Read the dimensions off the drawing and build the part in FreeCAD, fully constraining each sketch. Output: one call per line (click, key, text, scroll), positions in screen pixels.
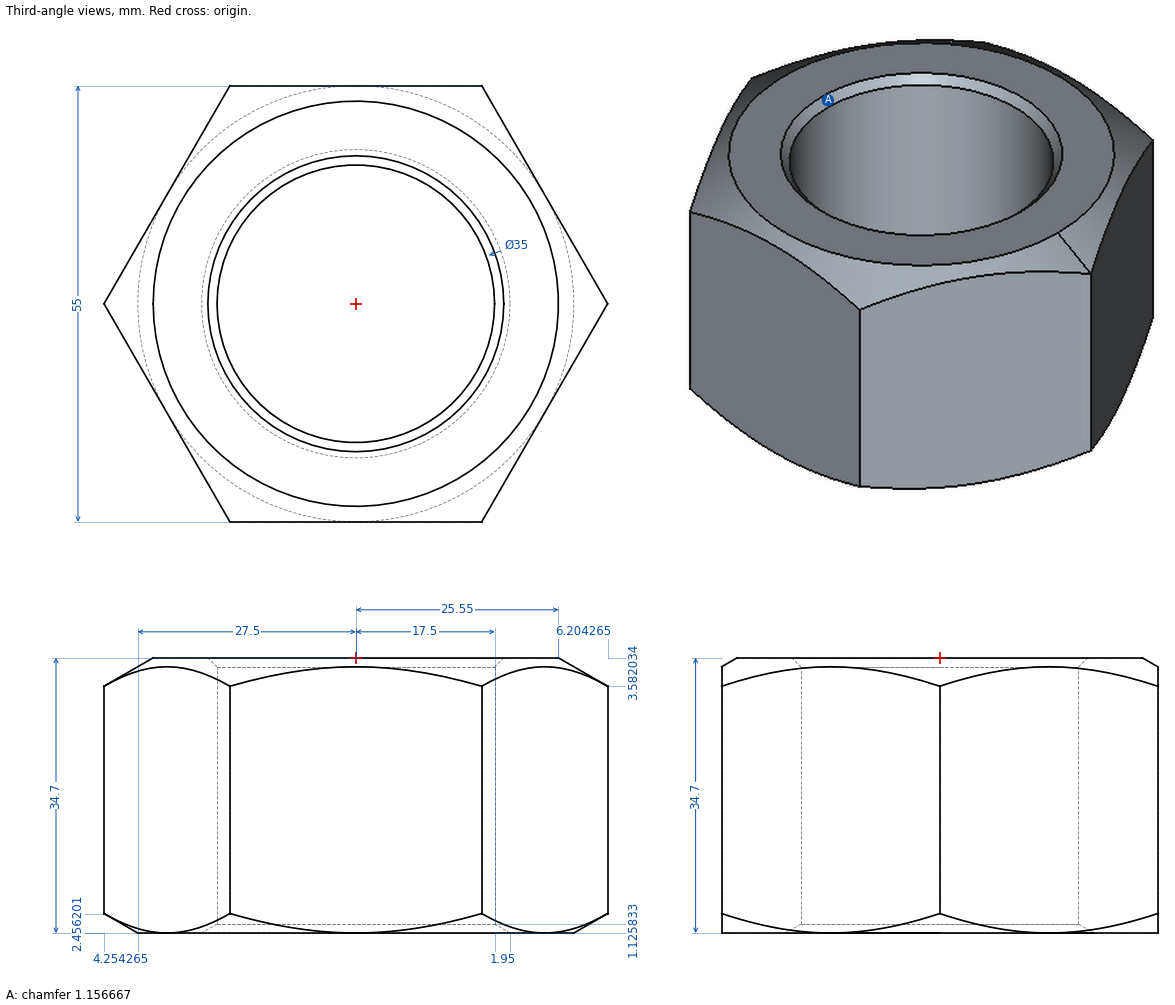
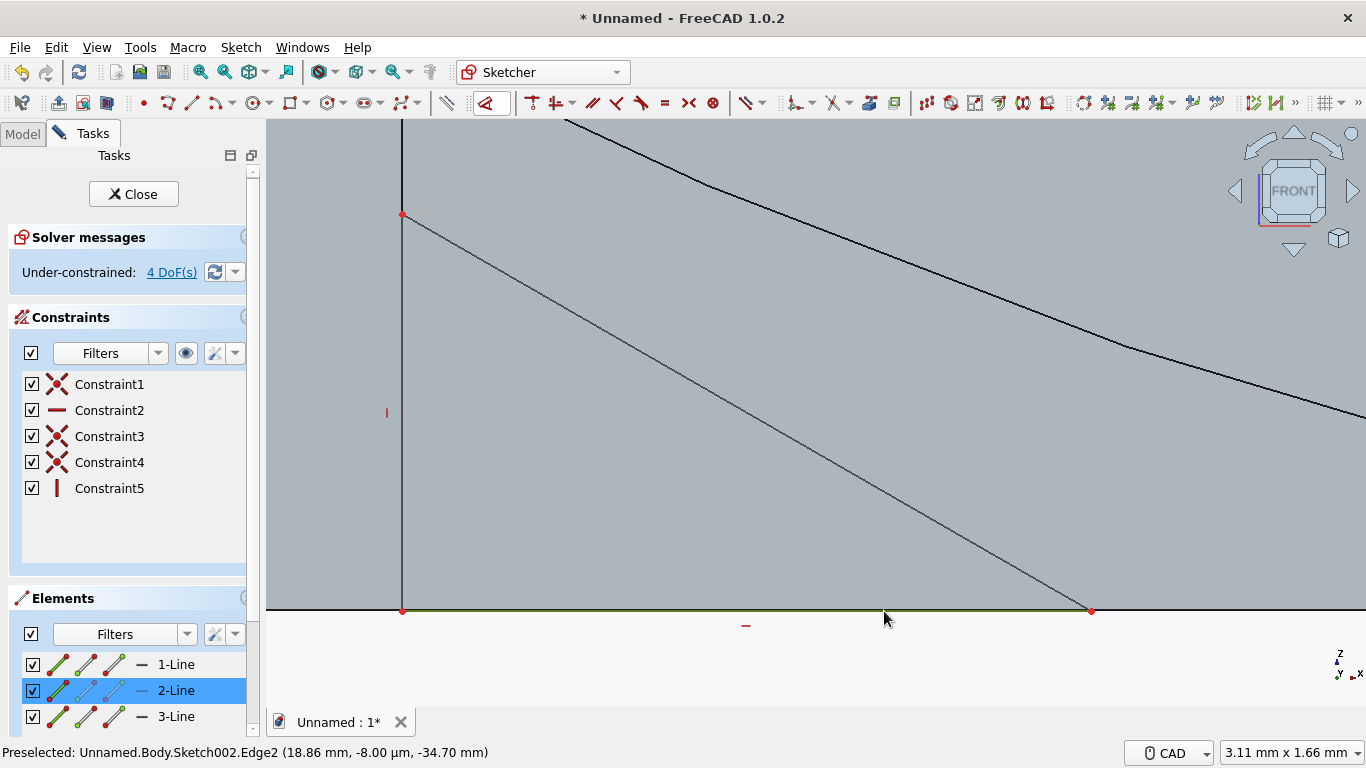
key(l)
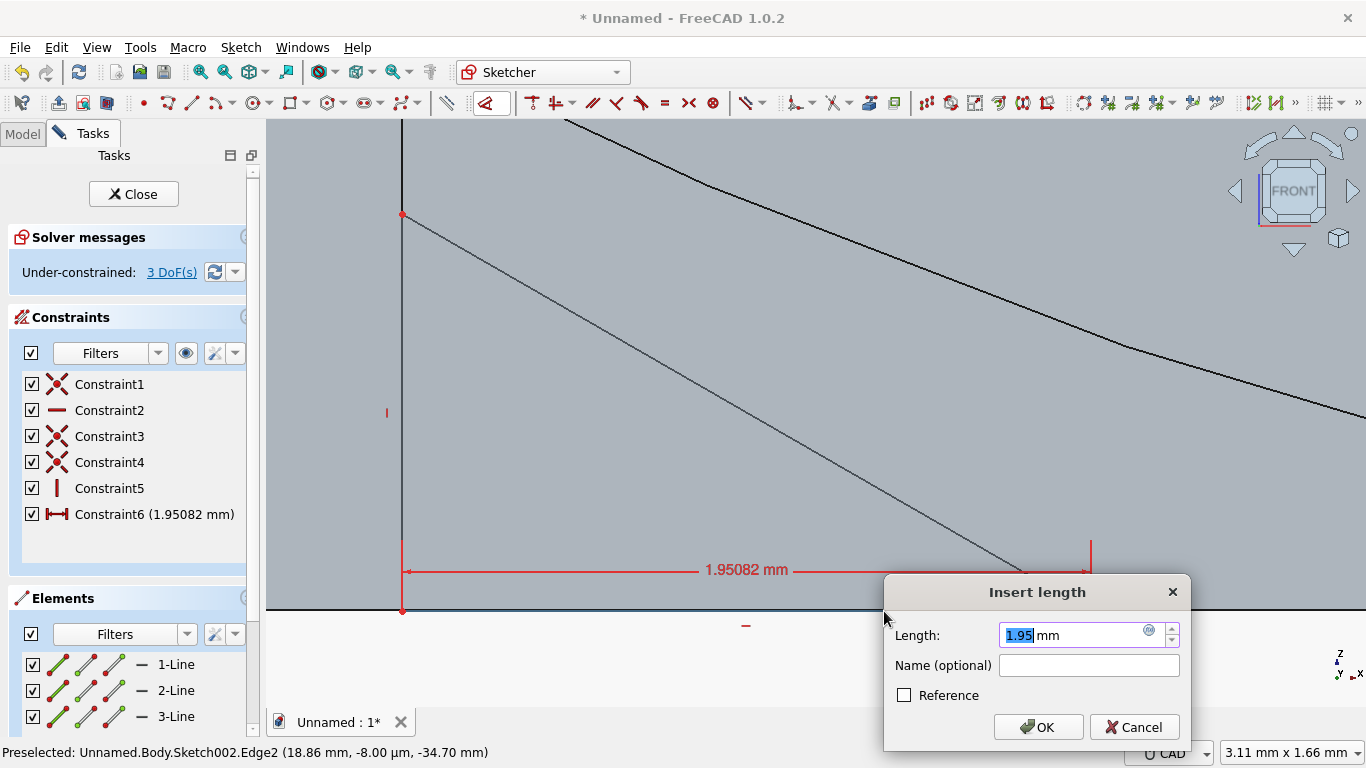
text(1.95)
key(Return)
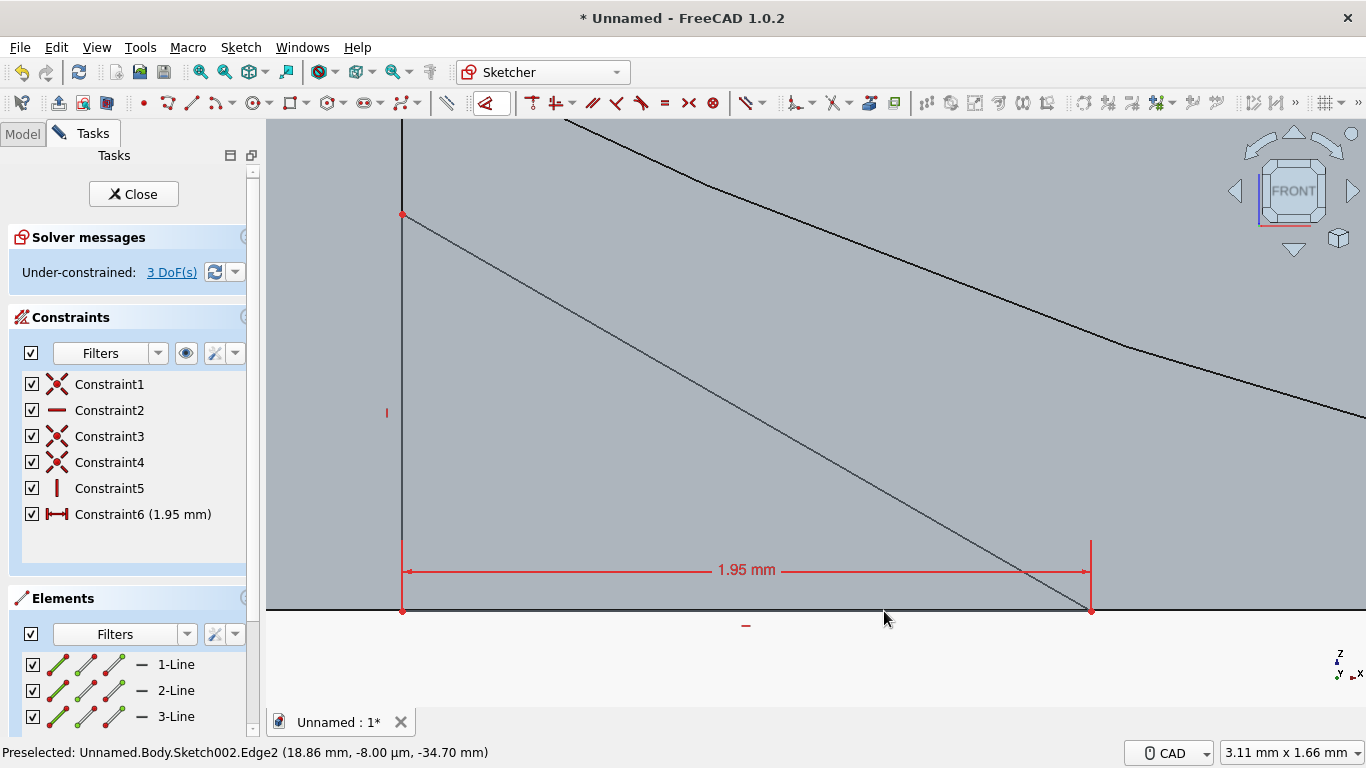
click(402, 214)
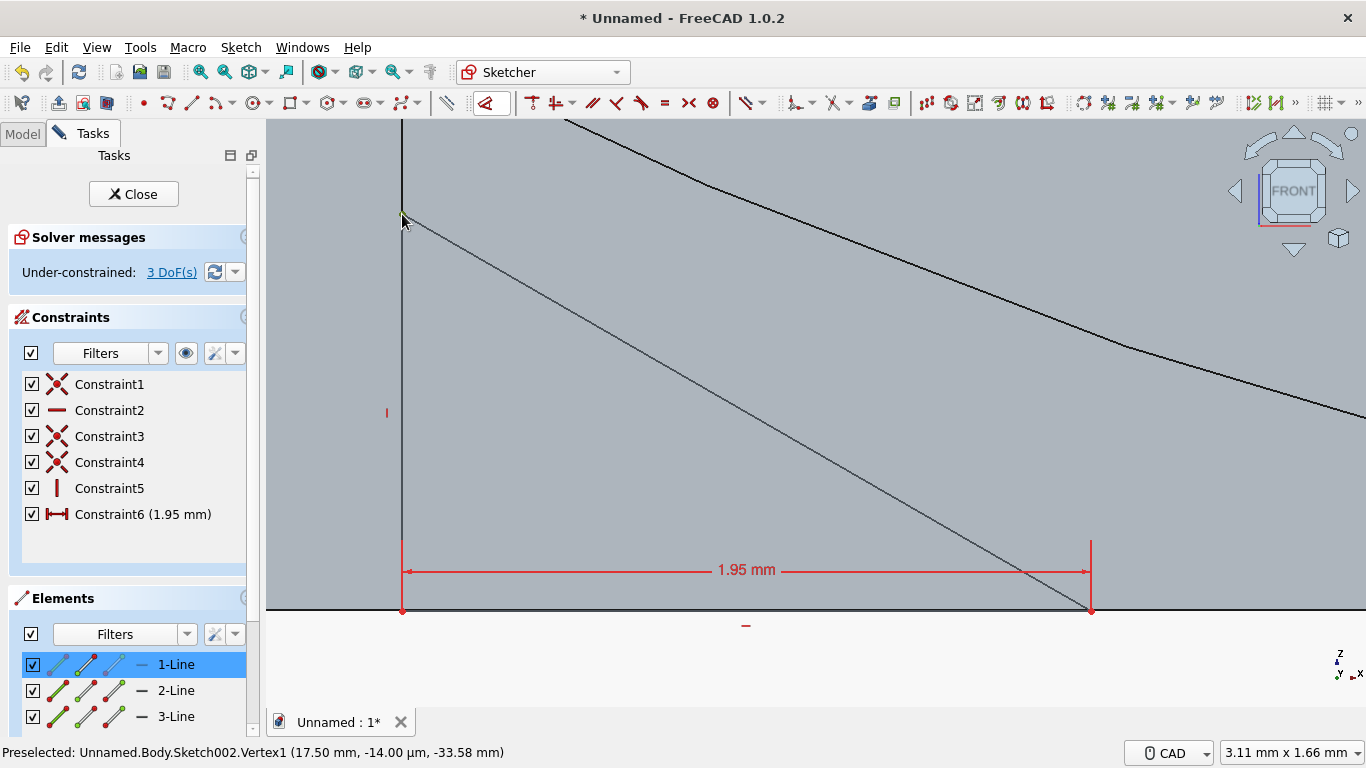
key(l)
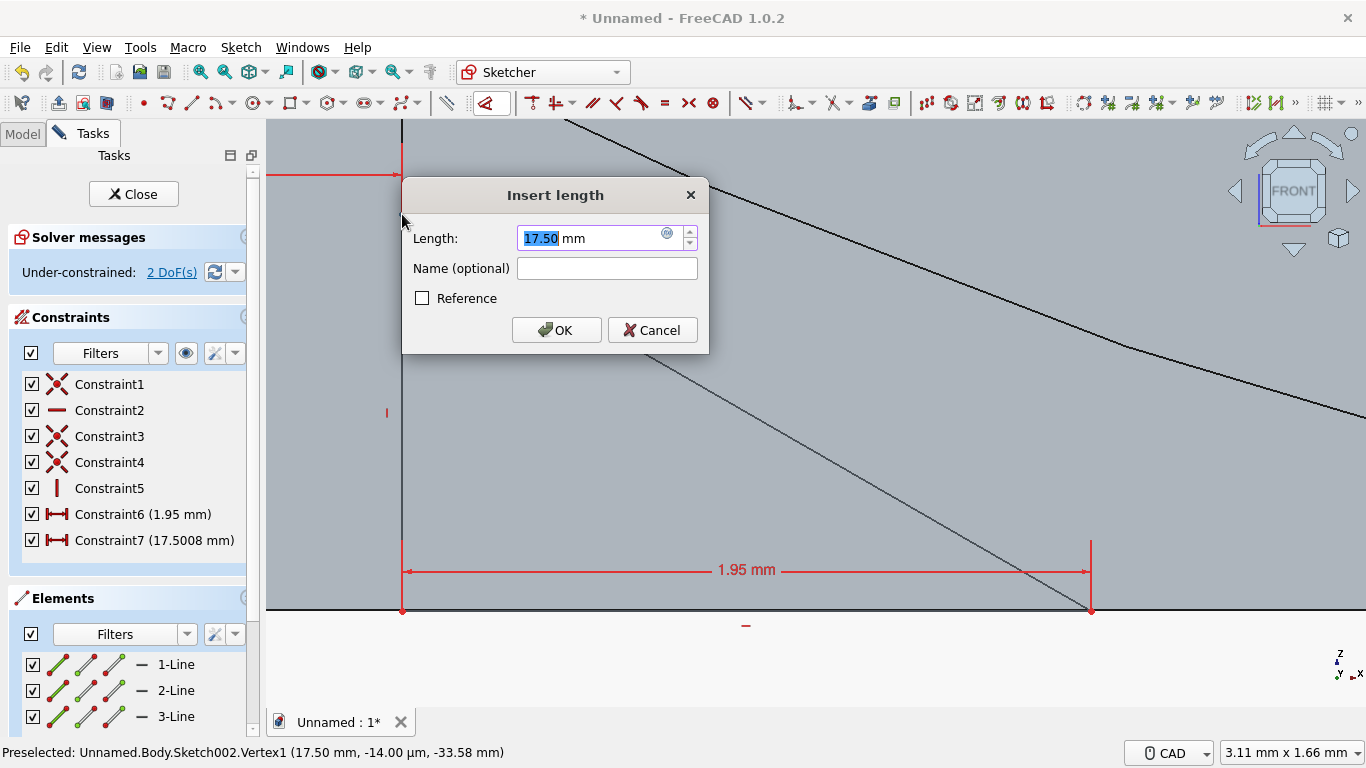
text(17.5)
key(Return)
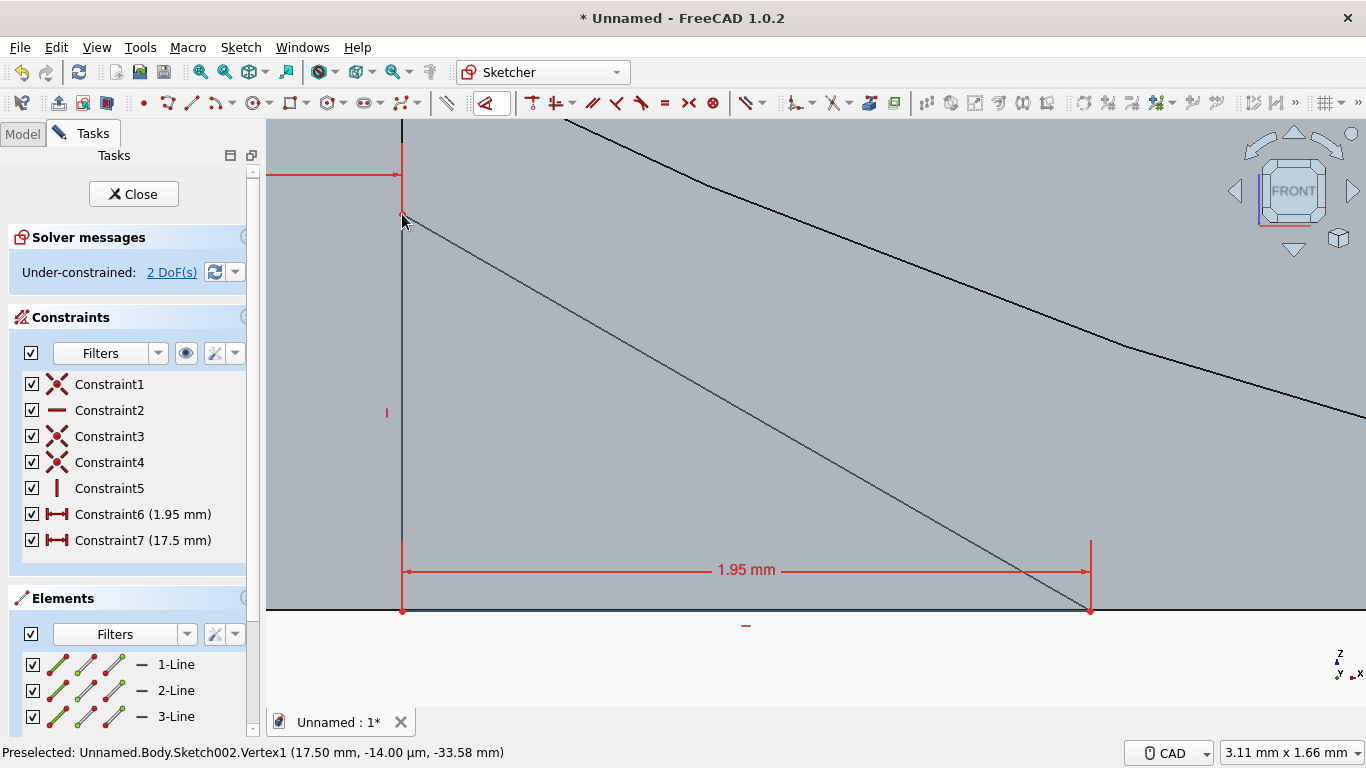
click(1091, 611)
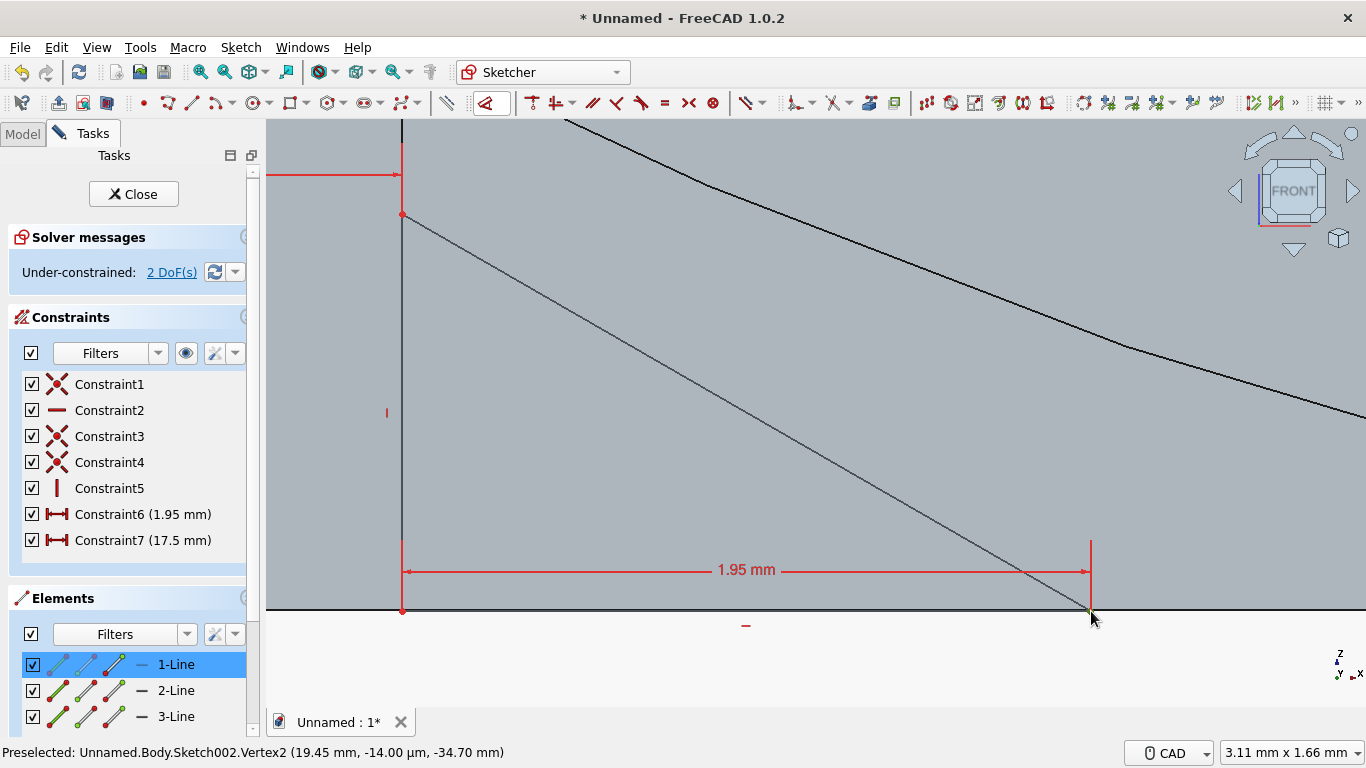
key(i)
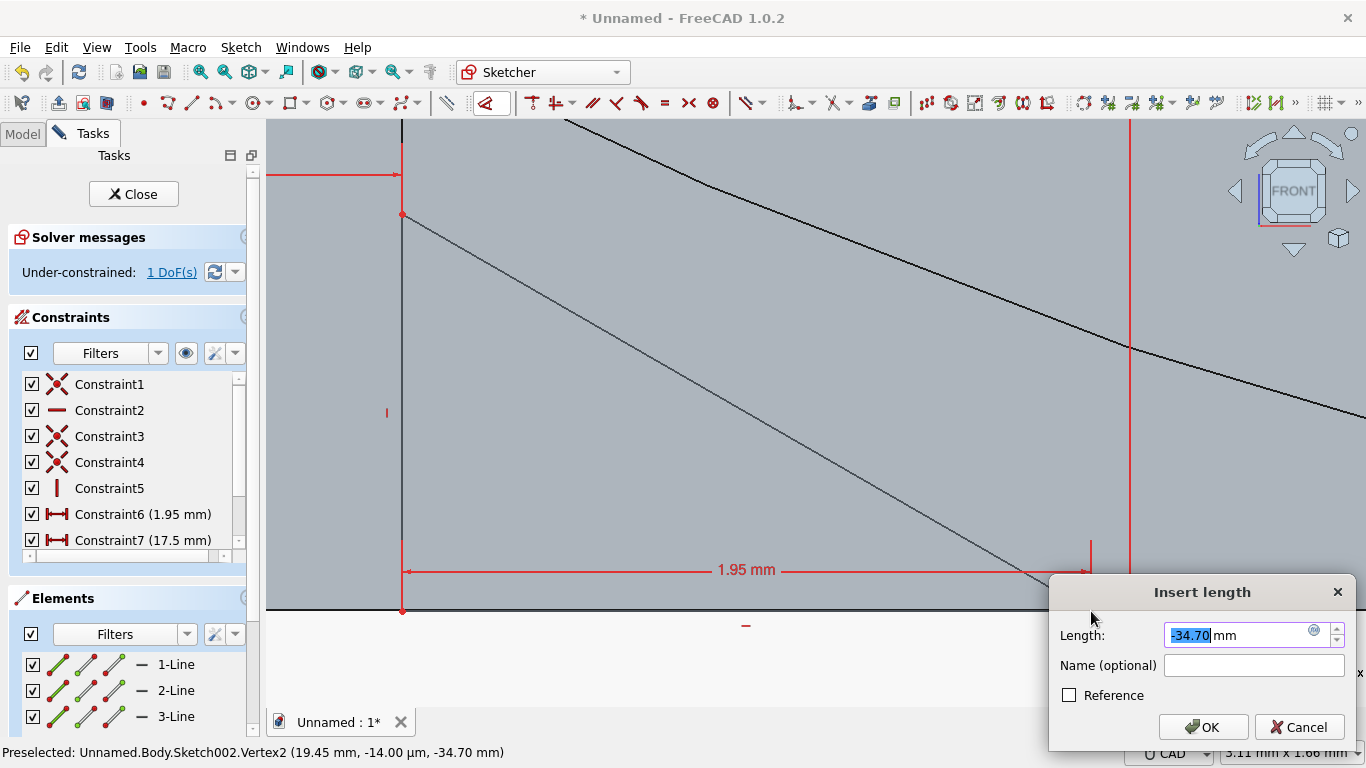
text(-34.7)
key(Return)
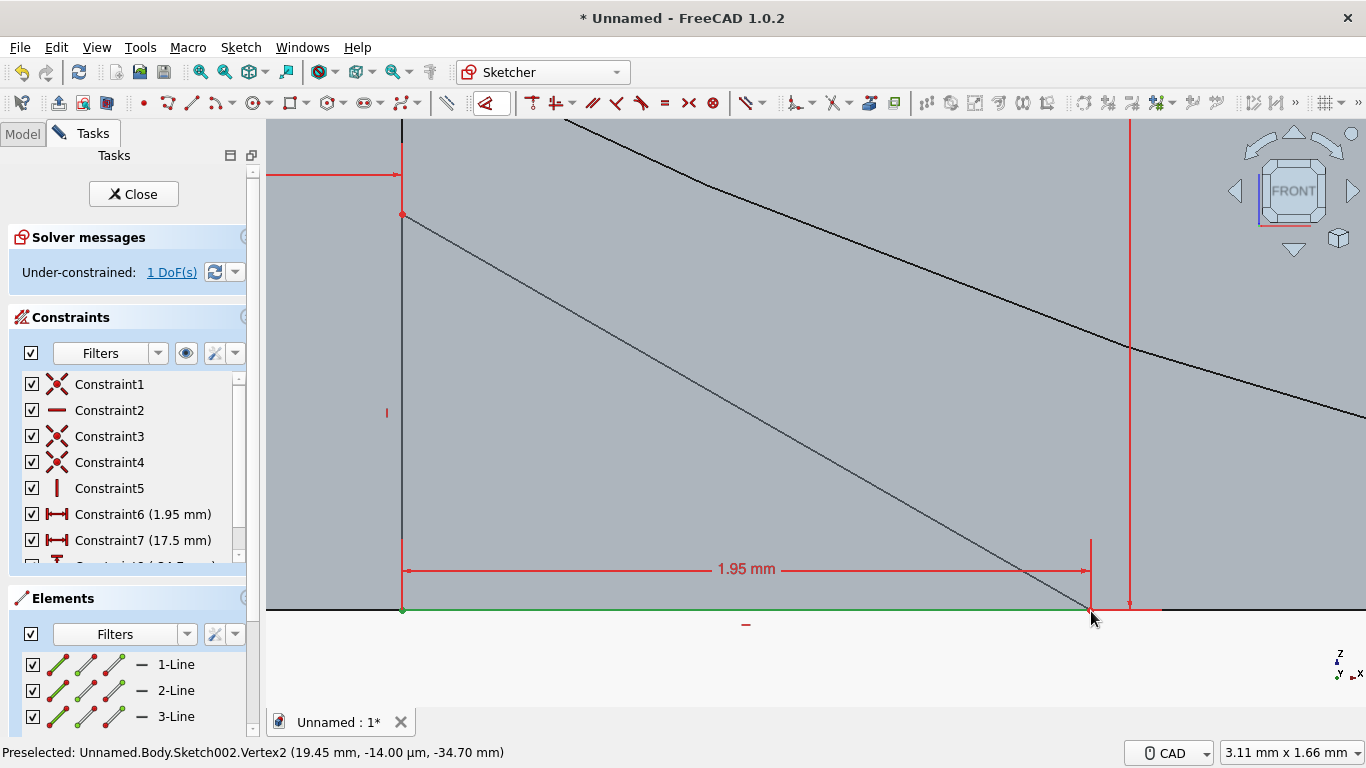
click(402, 491)